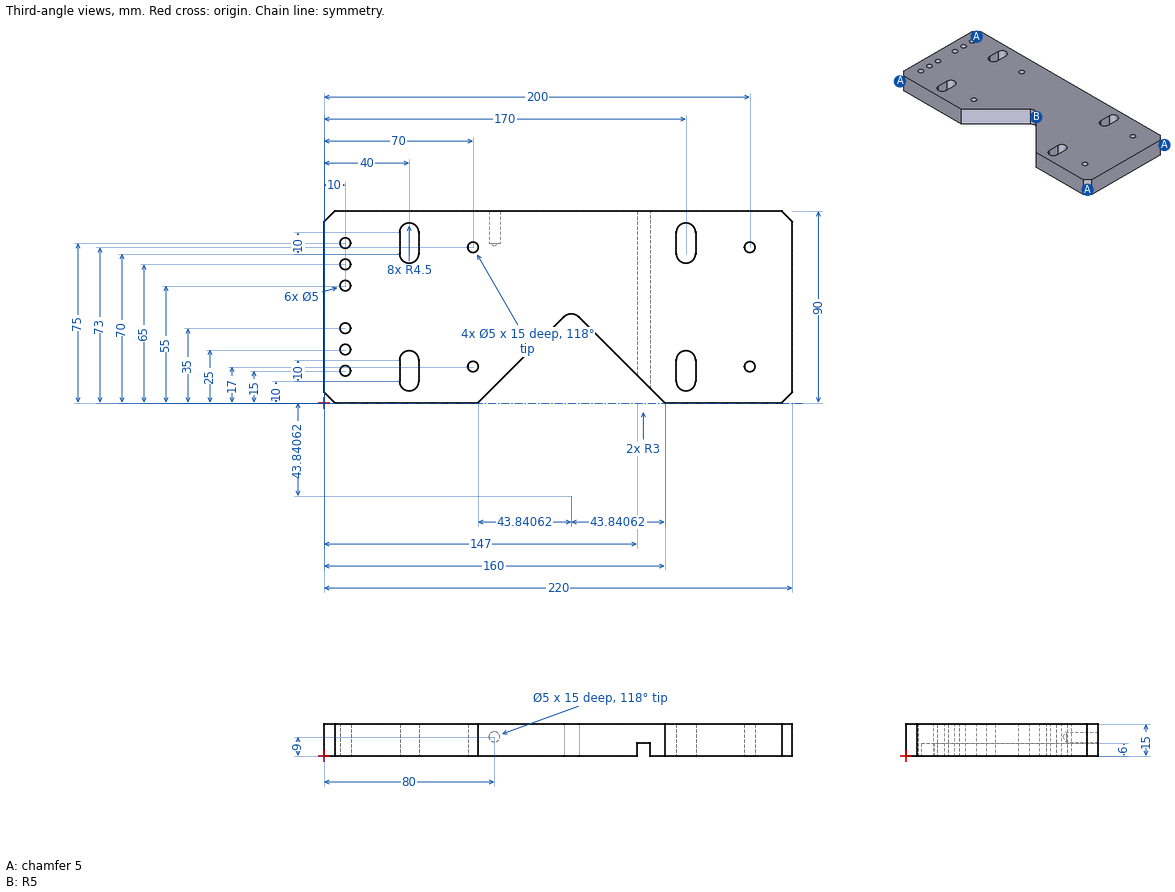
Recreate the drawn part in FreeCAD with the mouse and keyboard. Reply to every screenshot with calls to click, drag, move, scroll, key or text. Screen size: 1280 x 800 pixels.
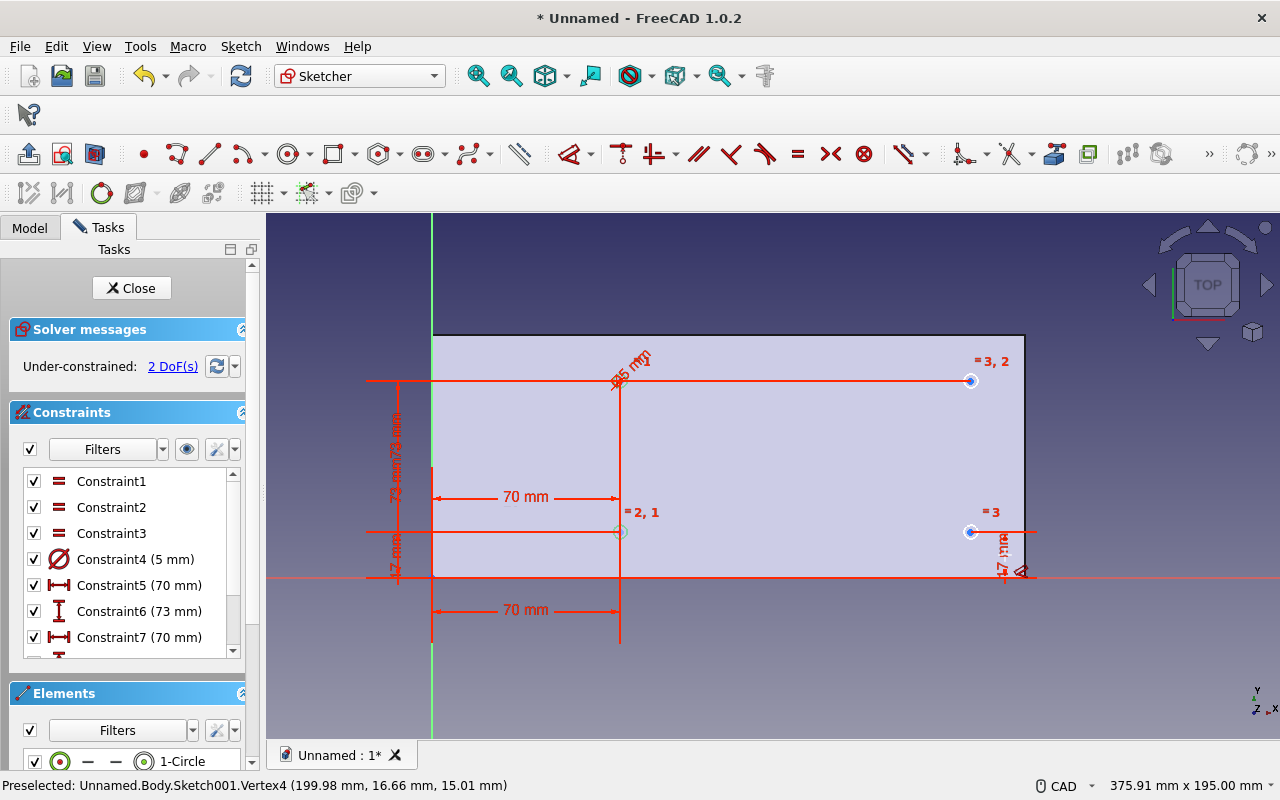
click(971, 381)
click(701, 612)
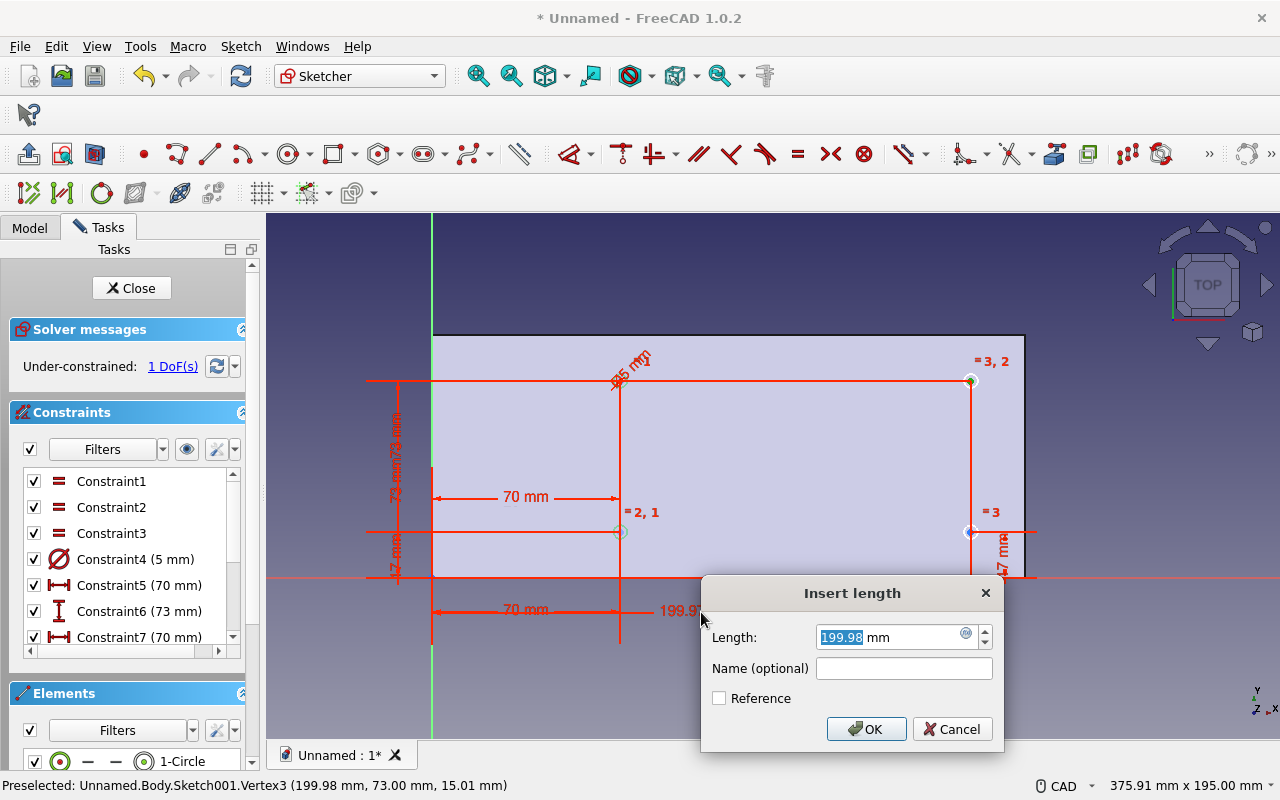
text(200)
key(Return)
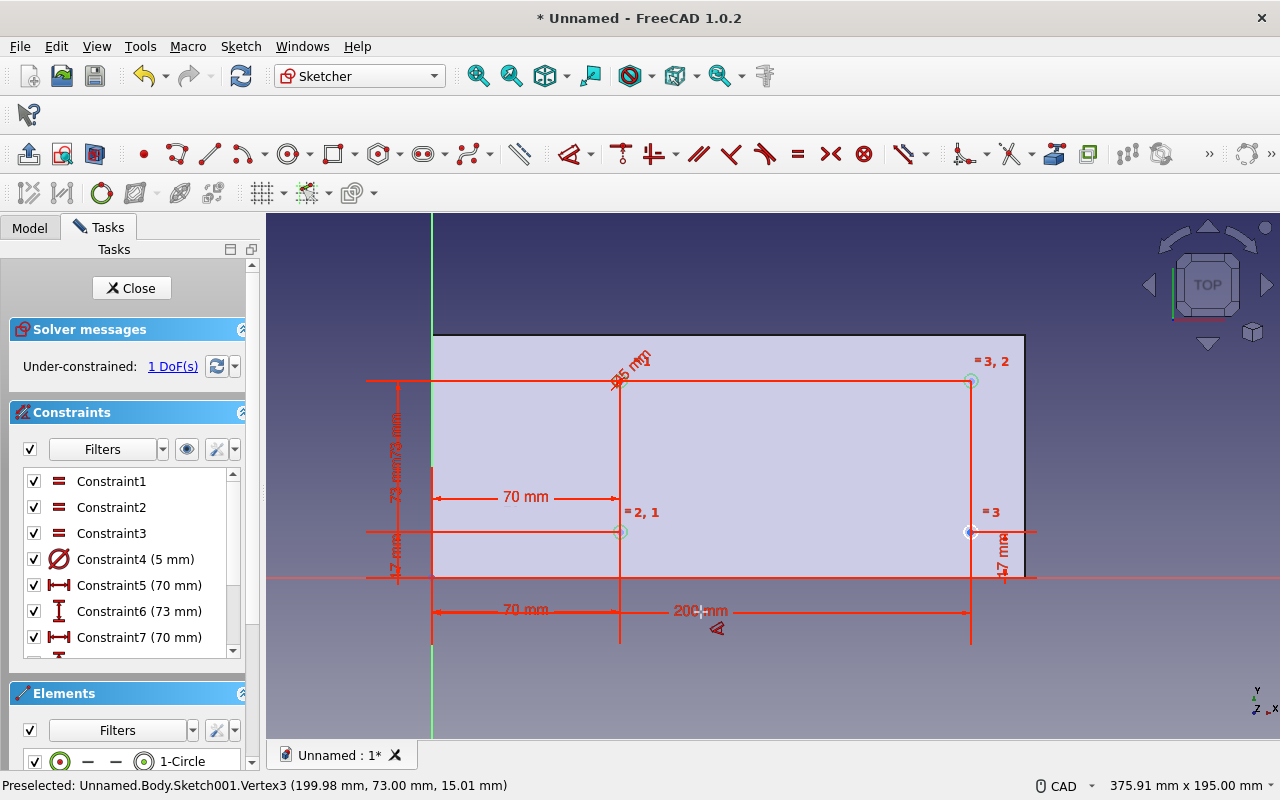
click(971, 532)
click(825, 612)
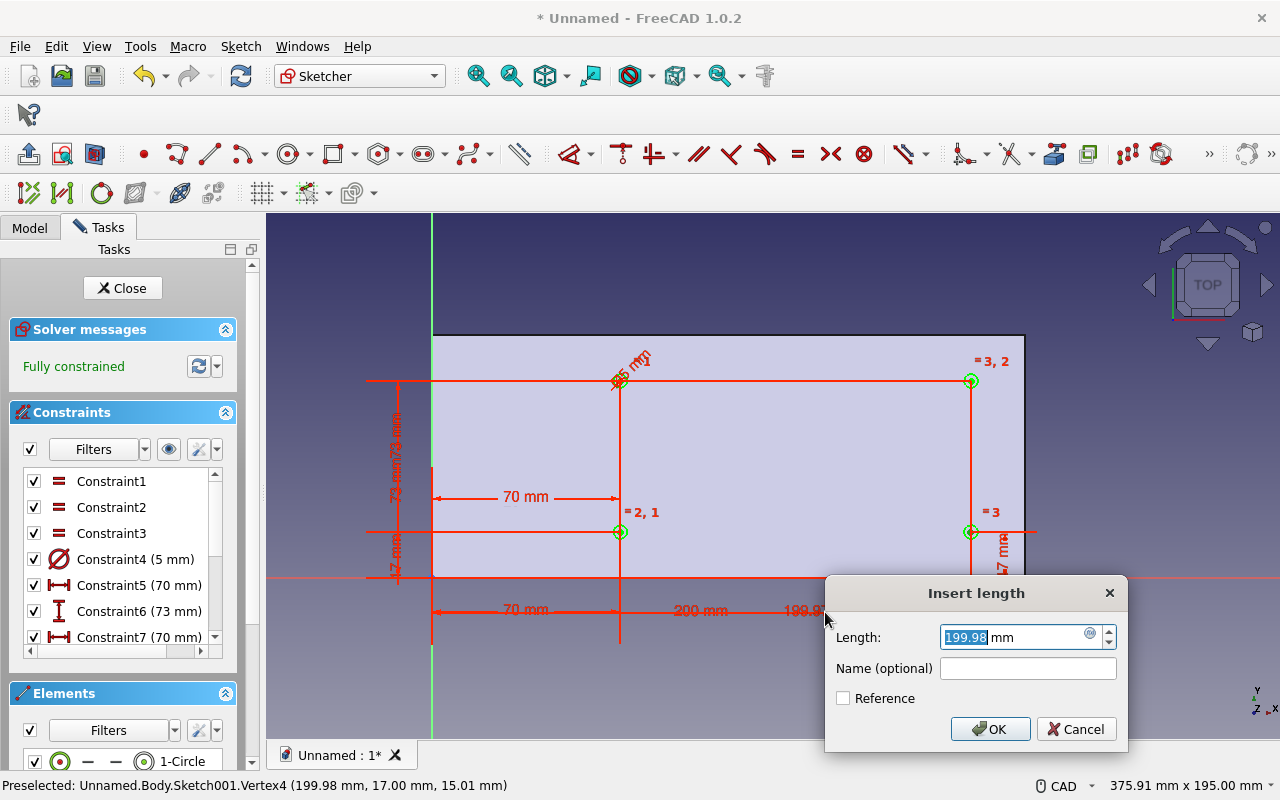
text(200)
key(Return)
key(Escape)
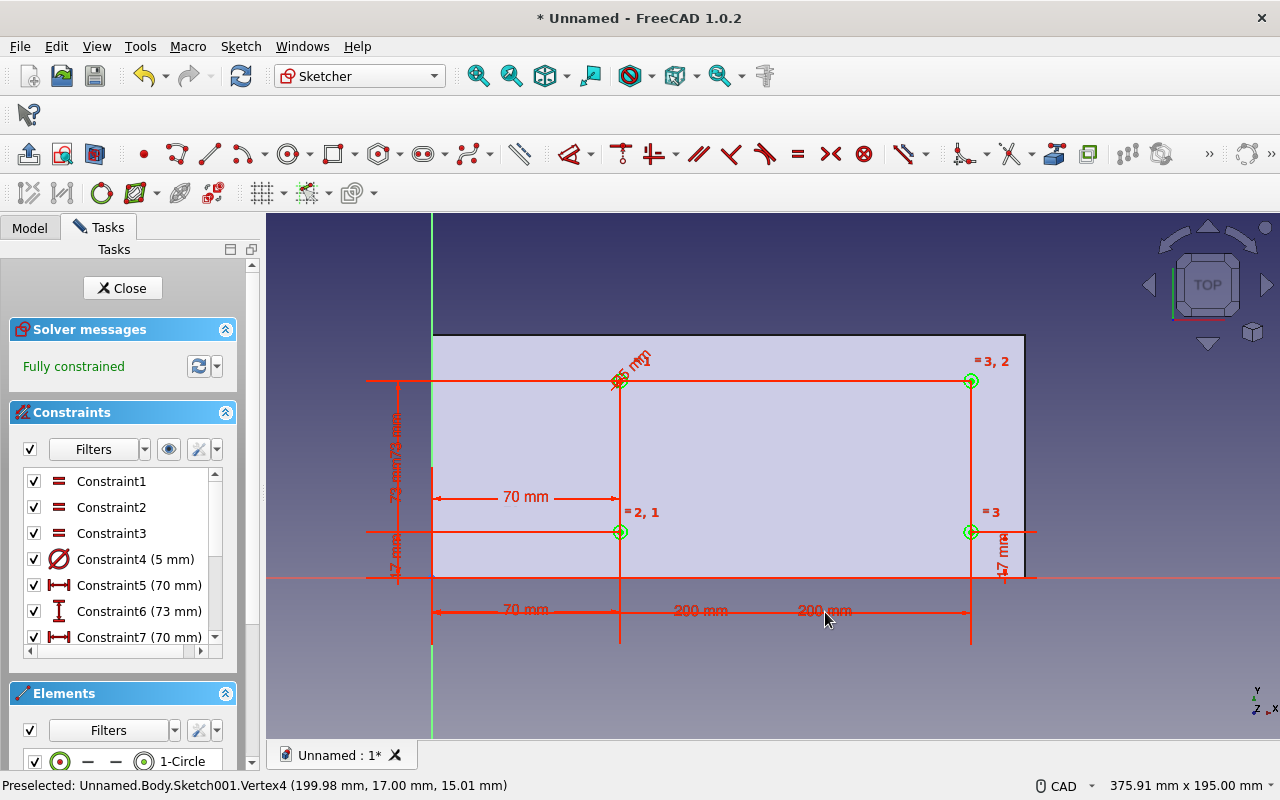
click(123, 288)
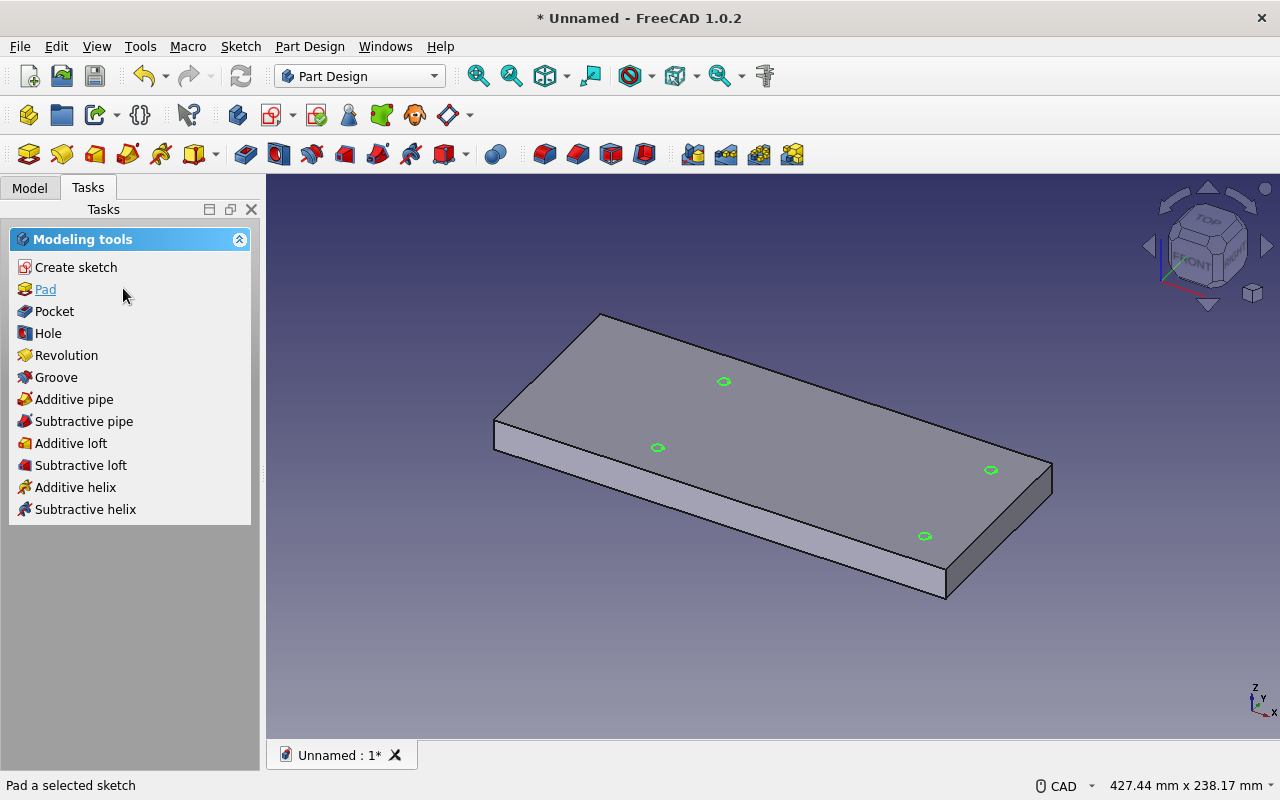
click(279, 154)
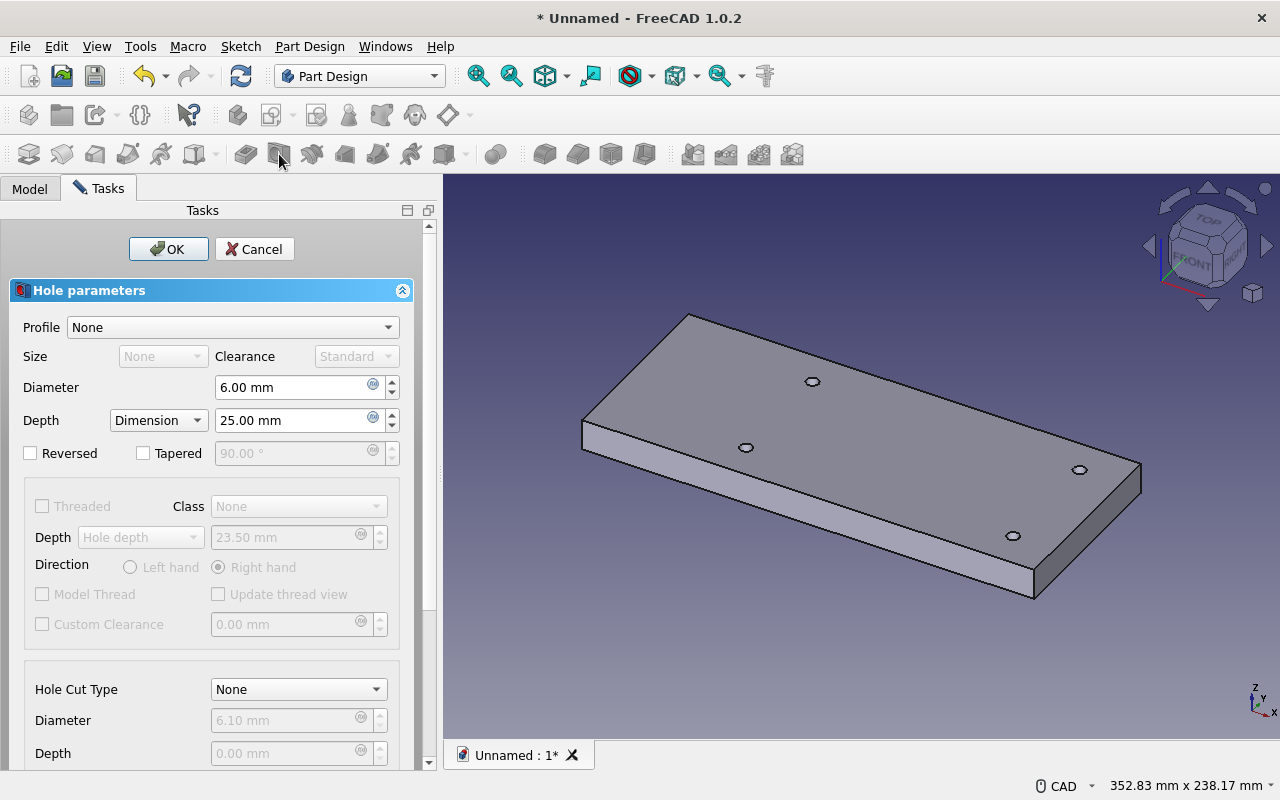
triple_click(300, 388)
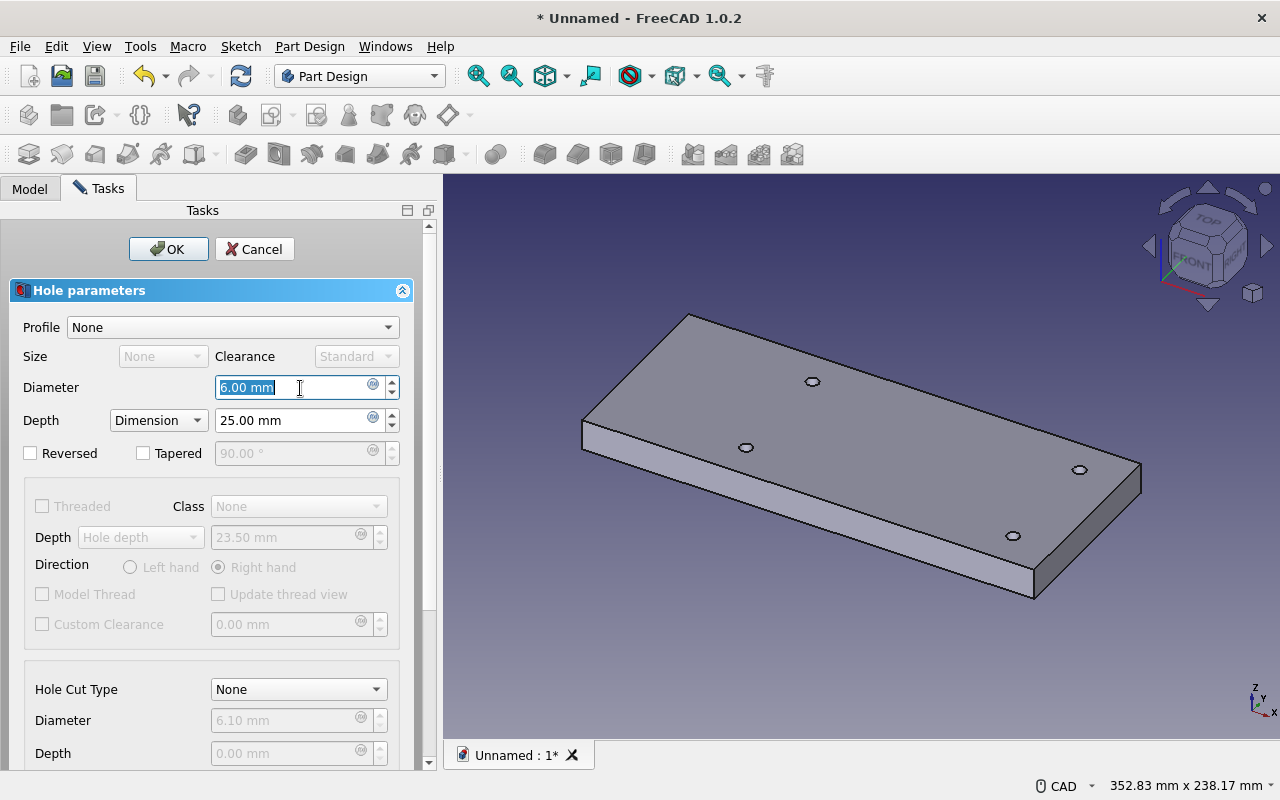
text(5)
key(Tab)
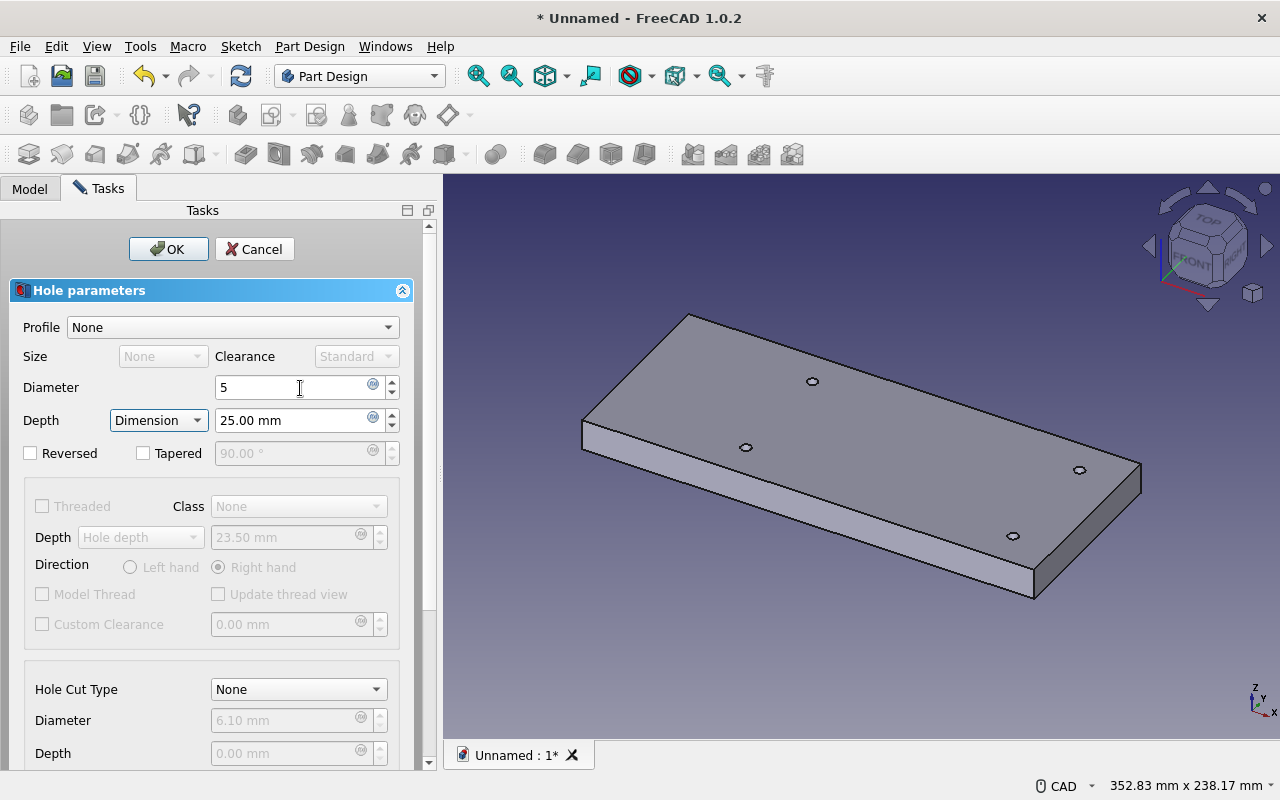
triple_click(300, 420)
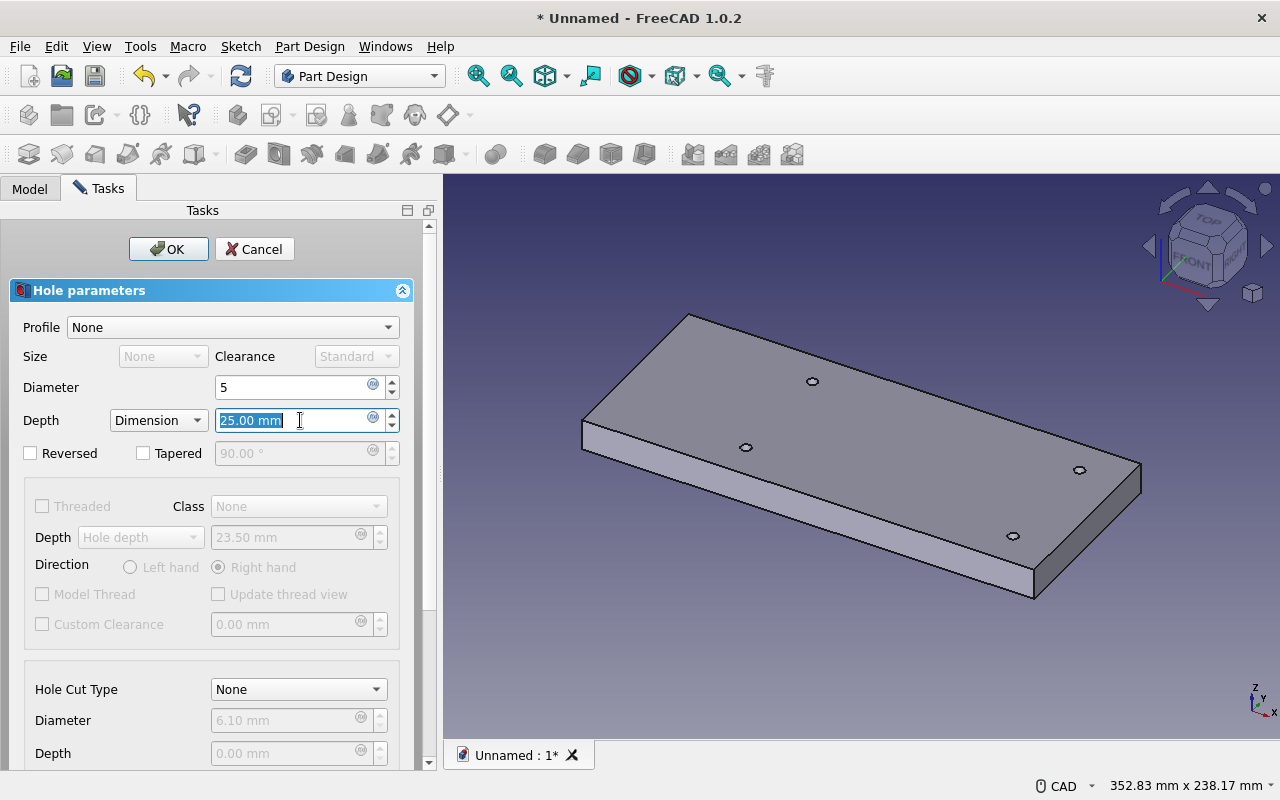
text(15)
key(Tab)